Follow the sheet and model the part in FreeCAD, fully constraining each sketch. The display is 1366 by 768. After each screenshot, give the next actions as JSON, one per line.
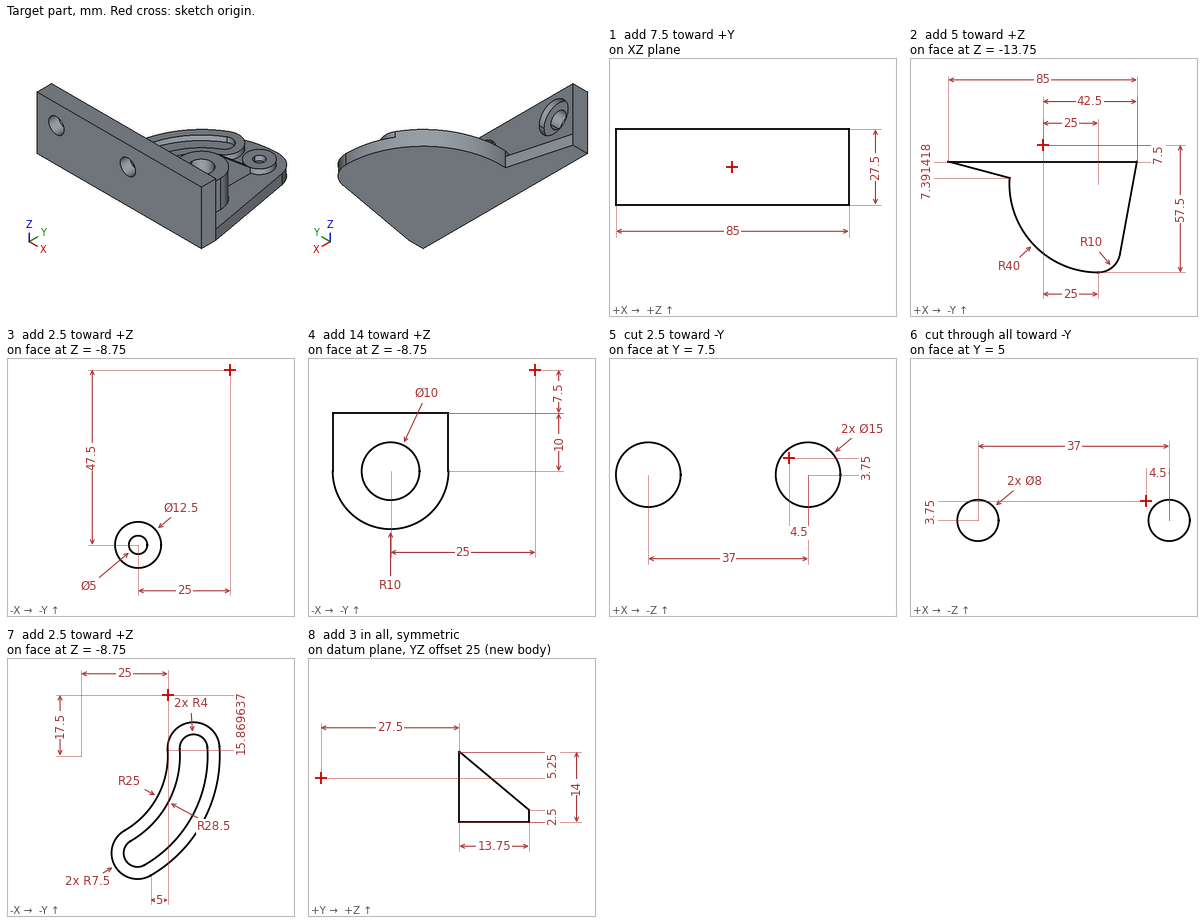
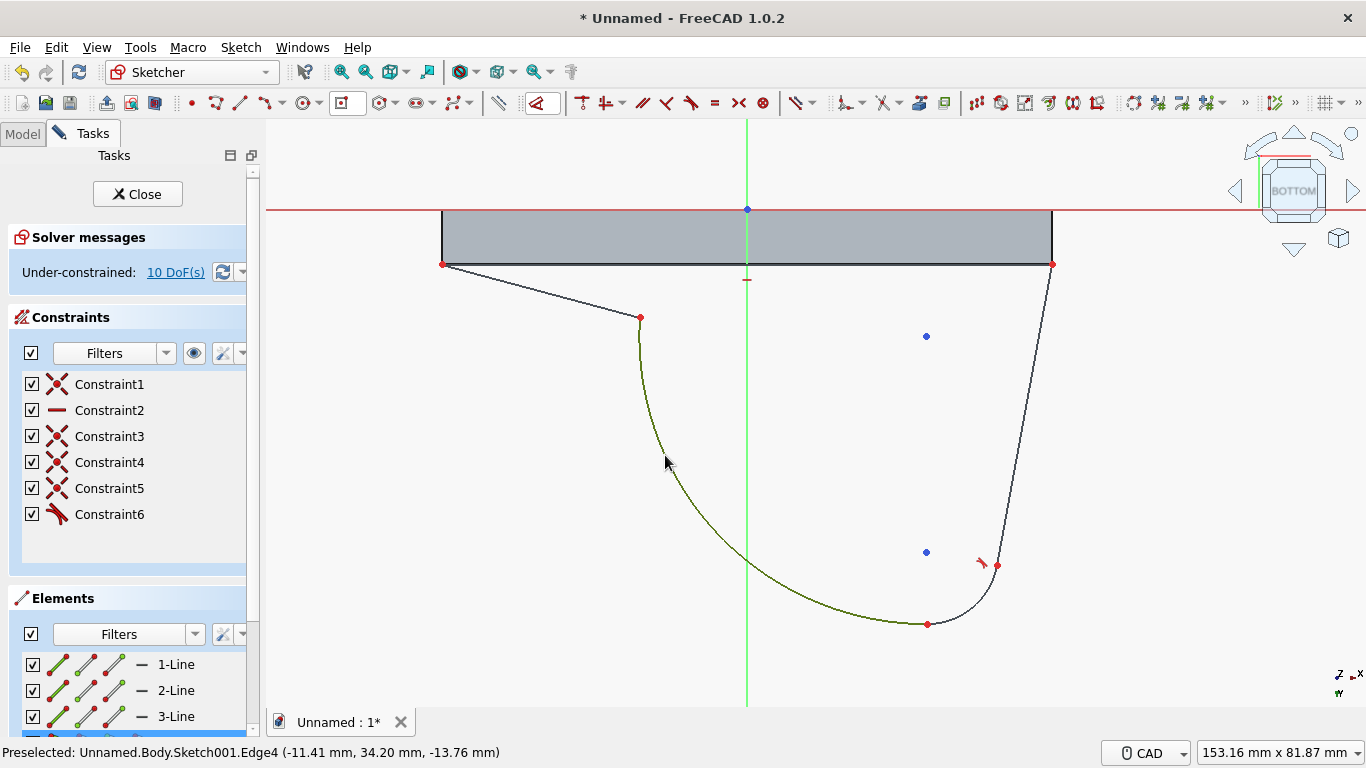
{"action": "left_click", "coordinate": [956, 618]}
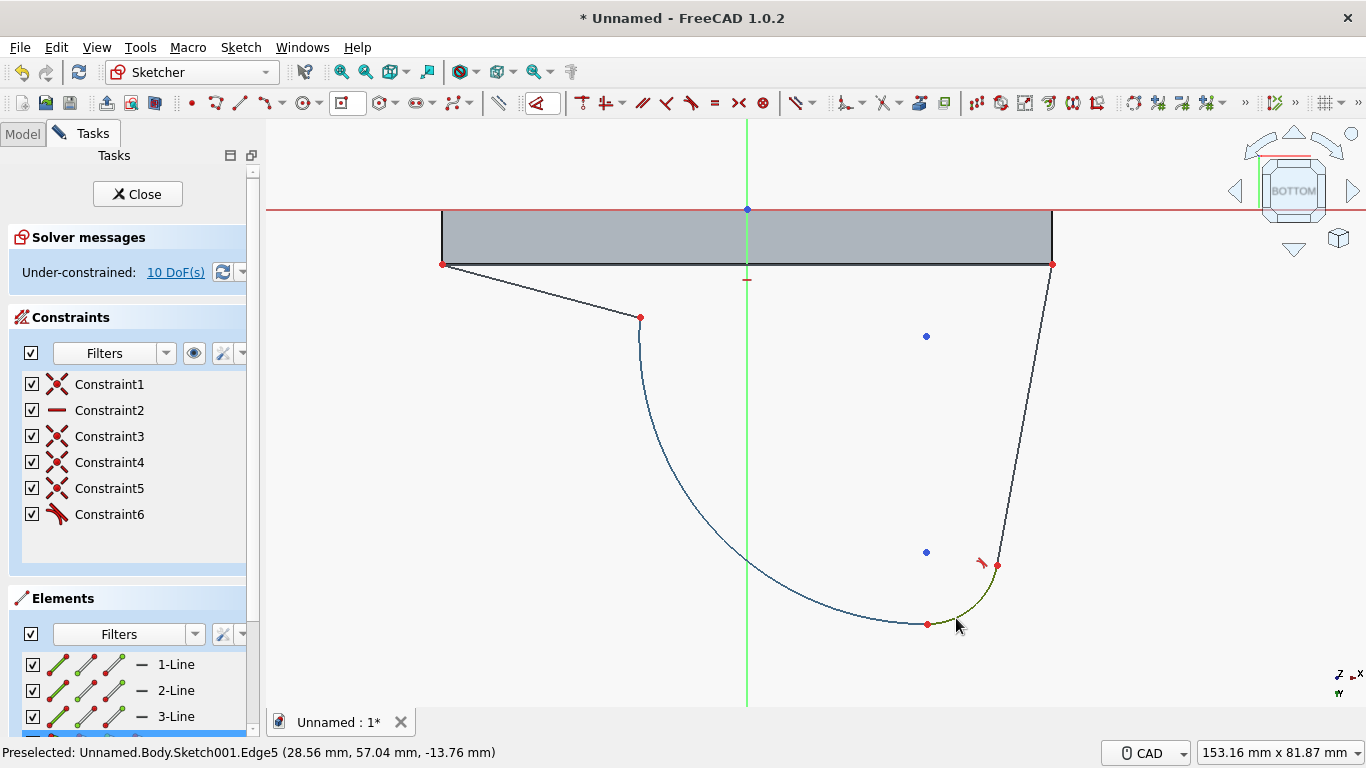
{"action": "left_click", "coordinate": [692, 104]}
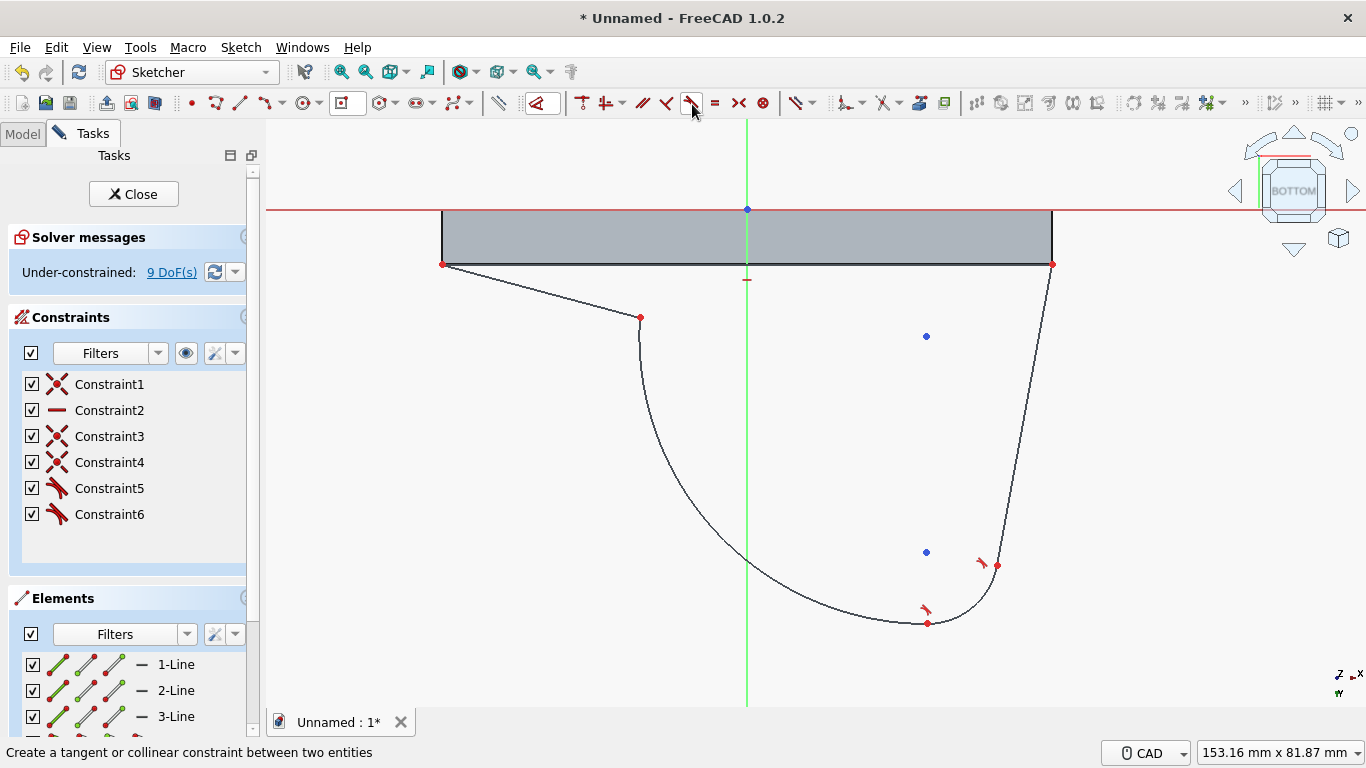
{"action": "left_click", "coordinate": [536, 104]}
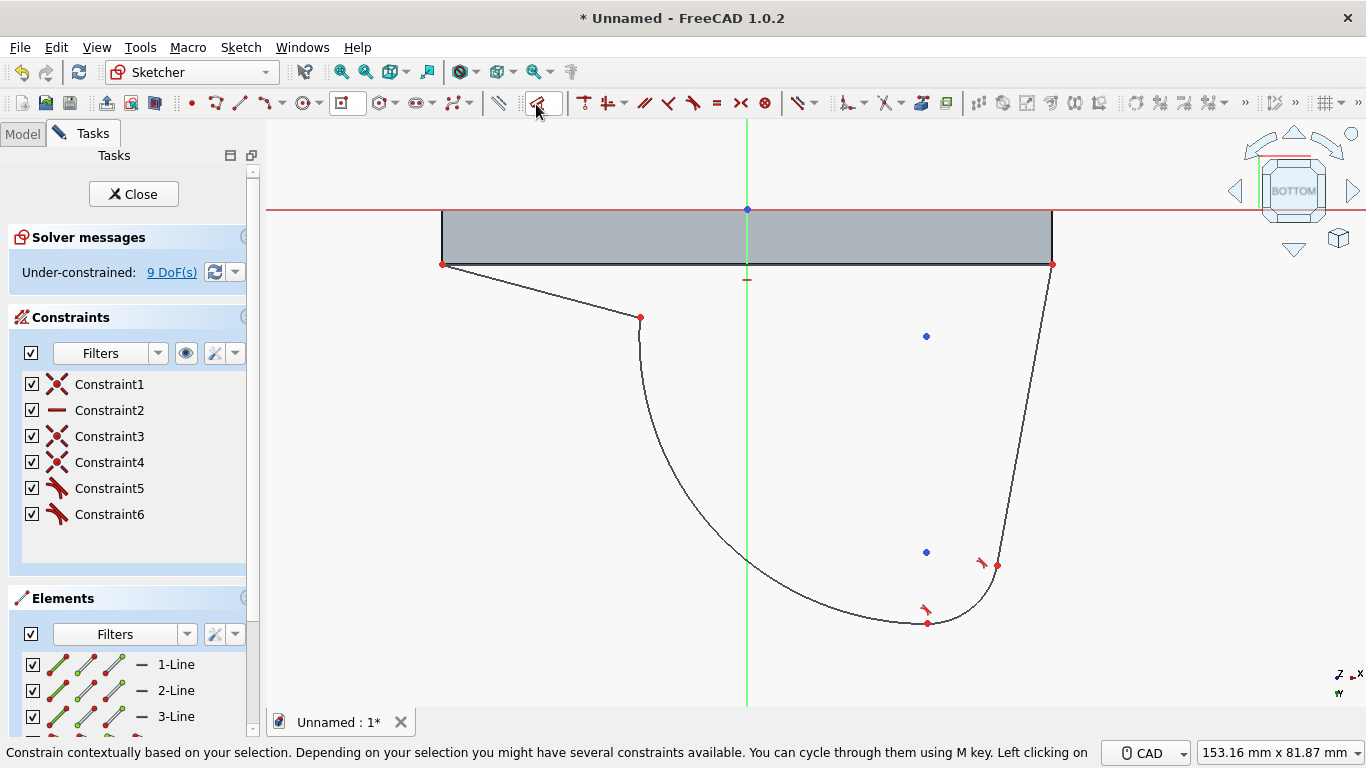
{"action": "left_click", "coordinate": [665, 455]}
{"action": "left_click", "coordinate": [636, 468]}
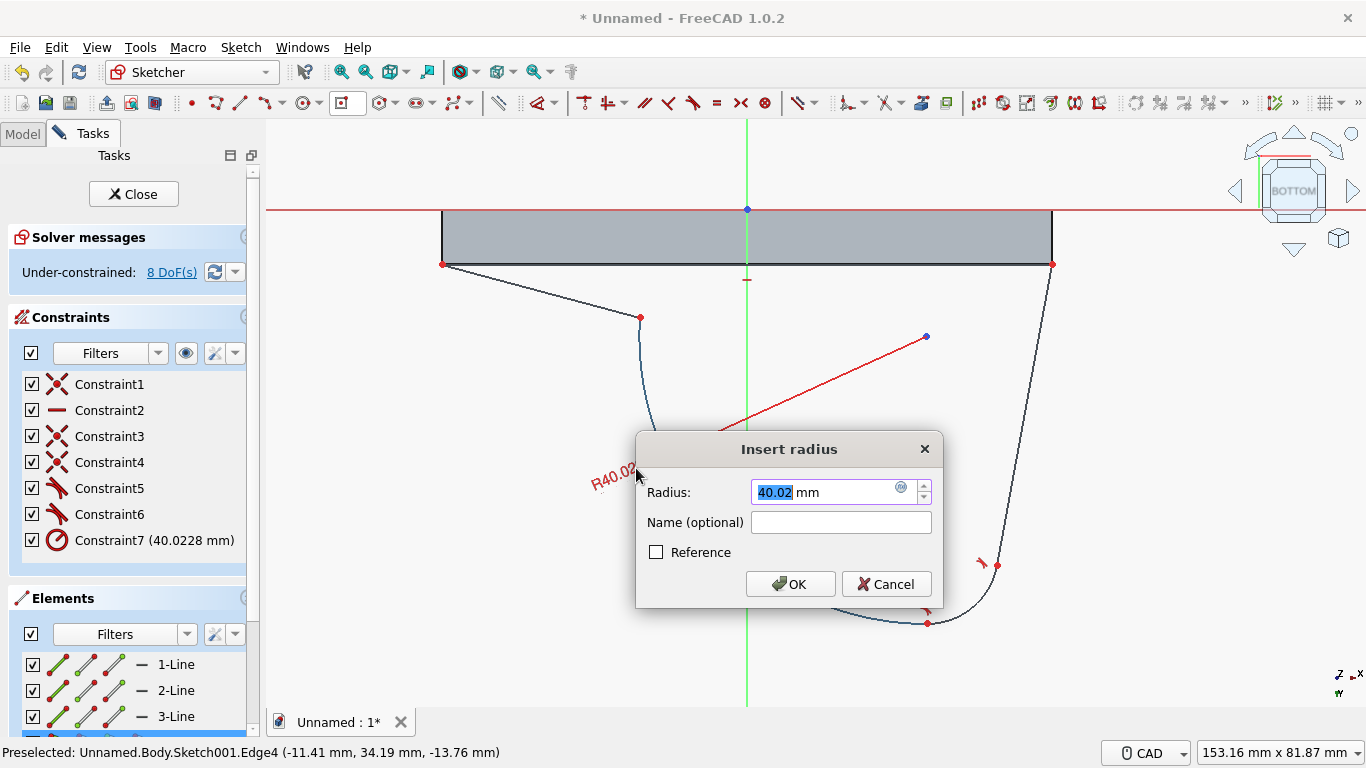
{"action": "type", "text": "40"}
{"action": "key", "text": "Return"}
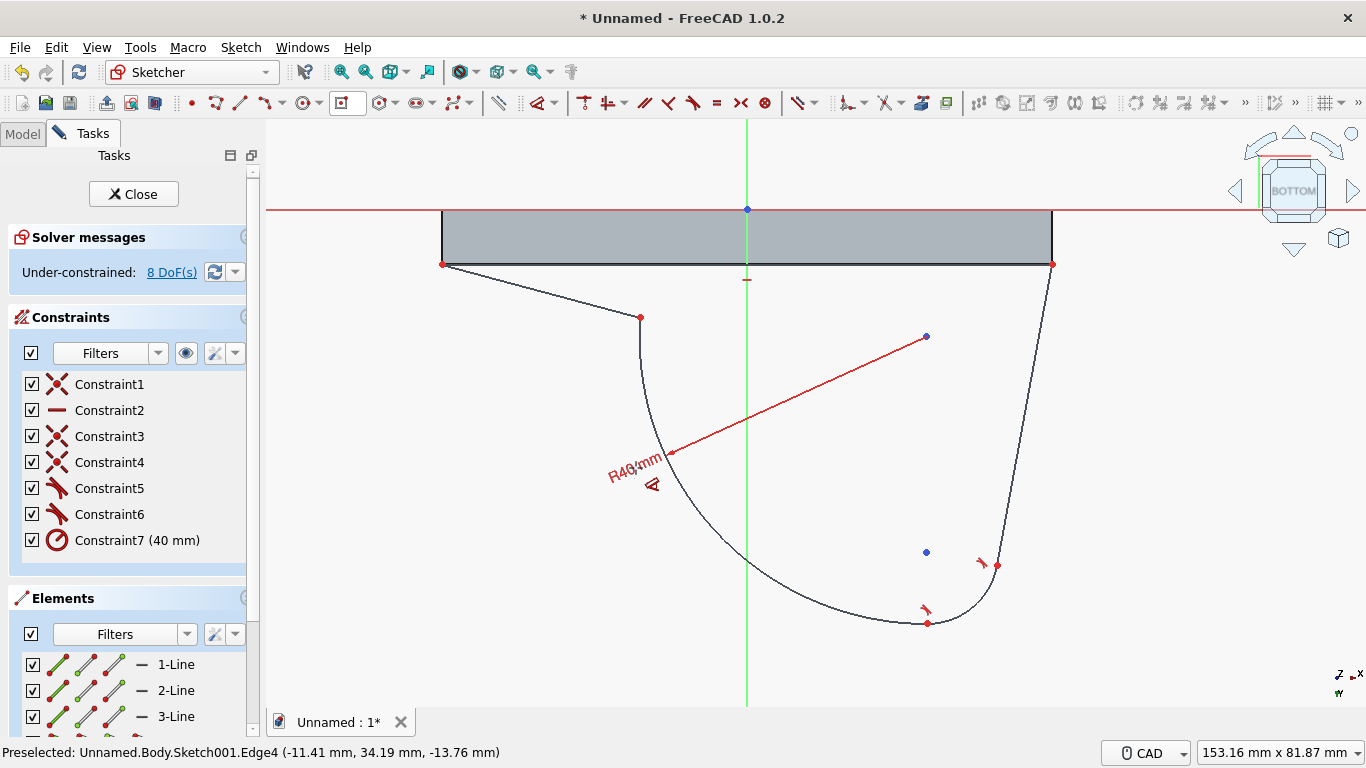
{"action": "left_click", "coordinate": [956, 618]}
{"action": "left_click", "coordinate": [969, 647]}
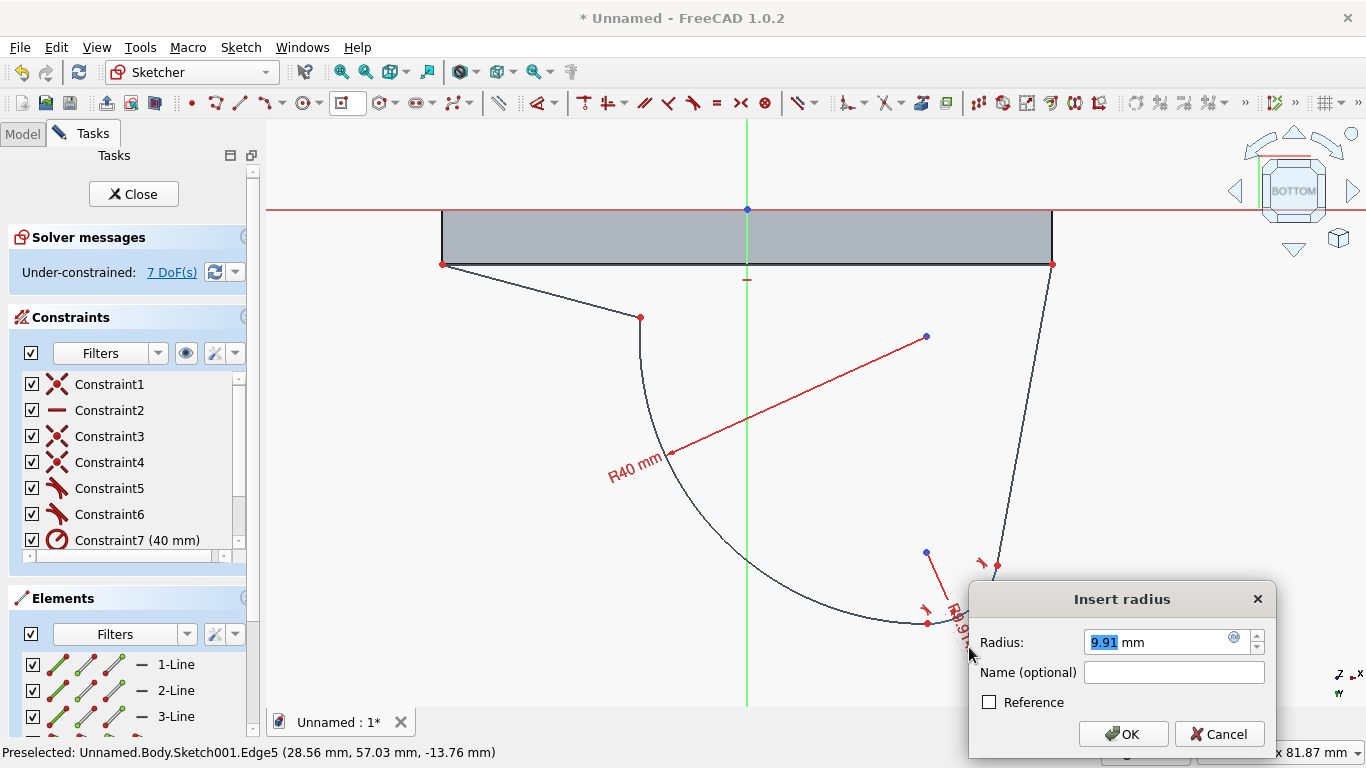
{"action": "type", "text": "10"}
{"action": "key", "text": "Return"}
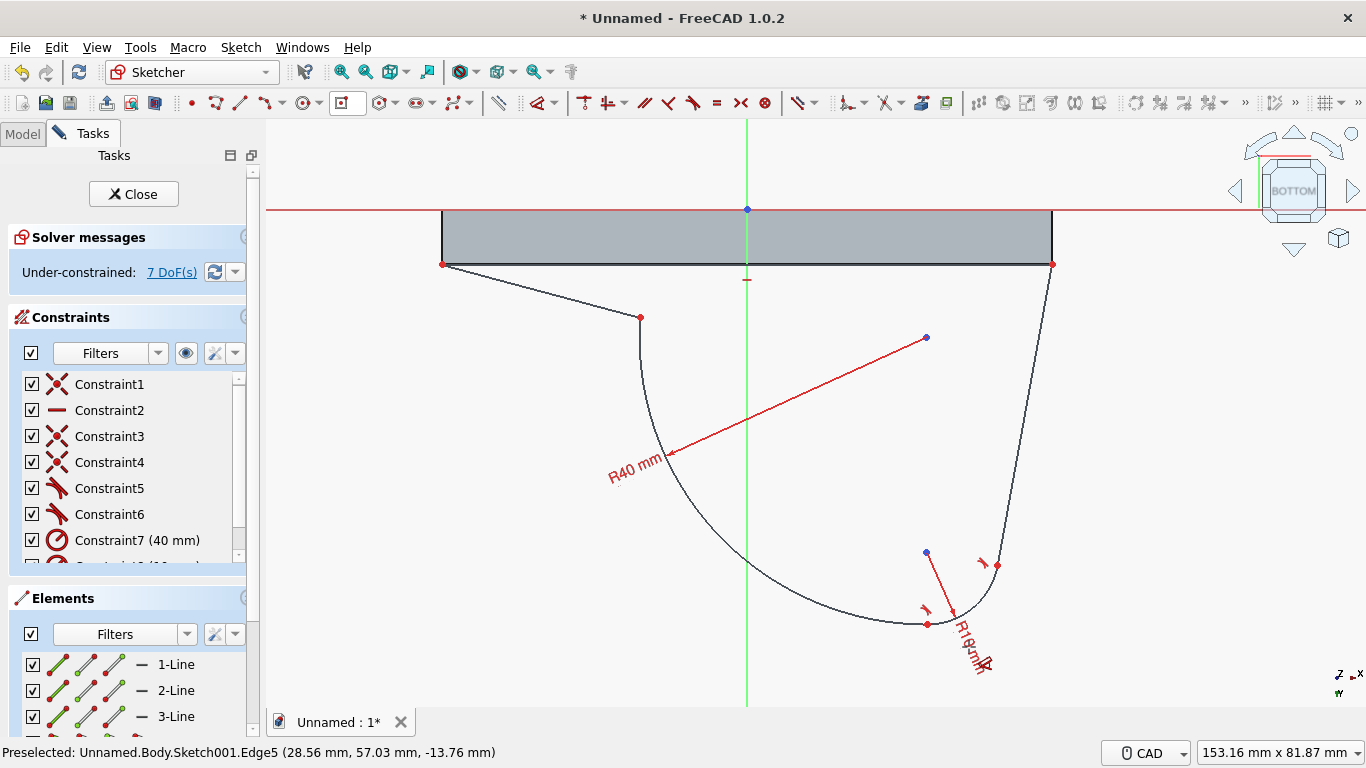
{"action": "left_click", "coordinate": [869, 265]}
{"action": "left_click", "coordinate": [607, 231]}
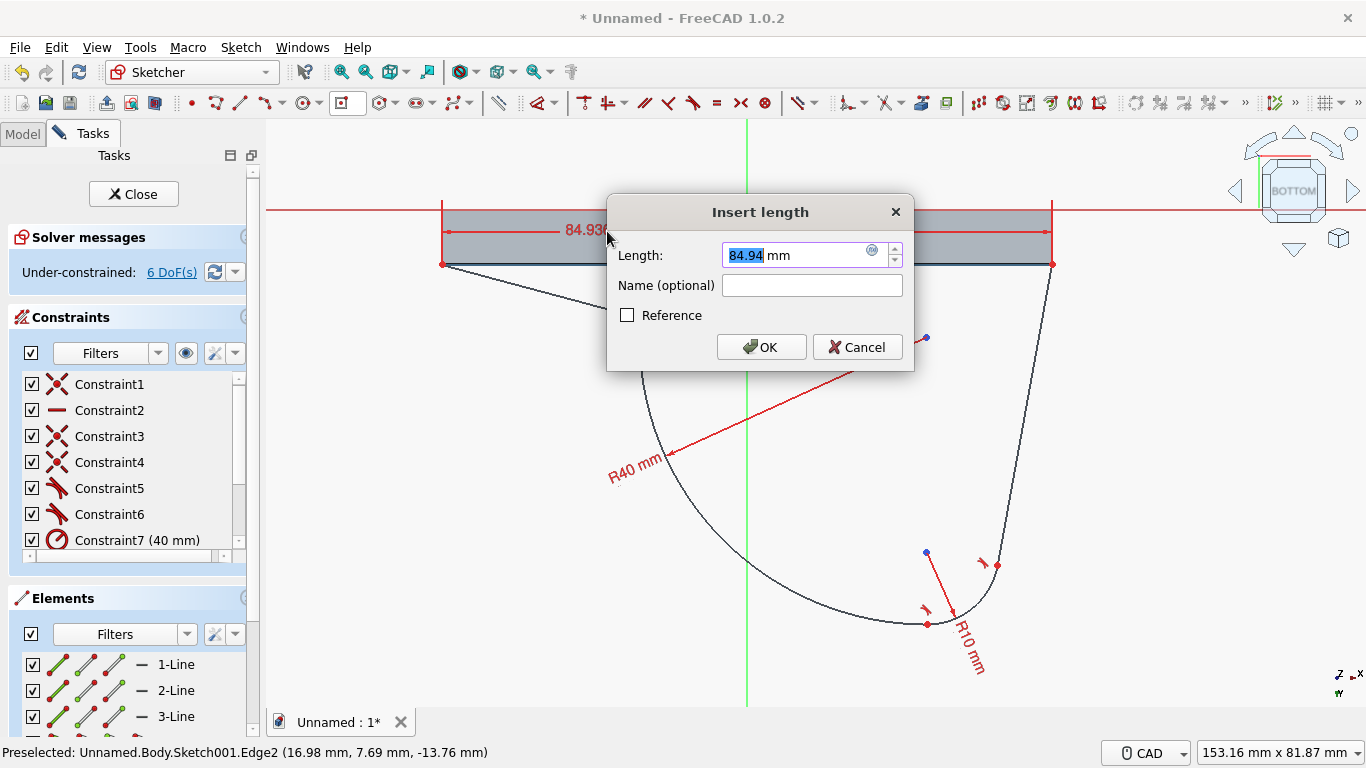
{"action": "type", "text": "85"}
{"action": "key", "text": "Return"}